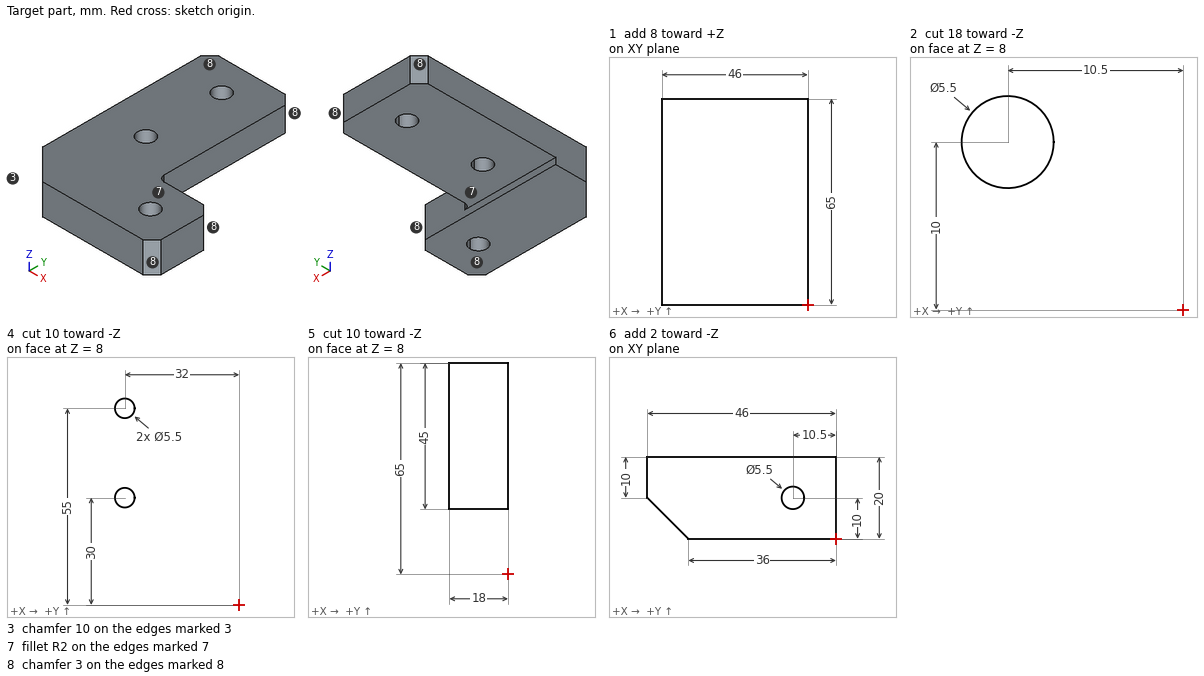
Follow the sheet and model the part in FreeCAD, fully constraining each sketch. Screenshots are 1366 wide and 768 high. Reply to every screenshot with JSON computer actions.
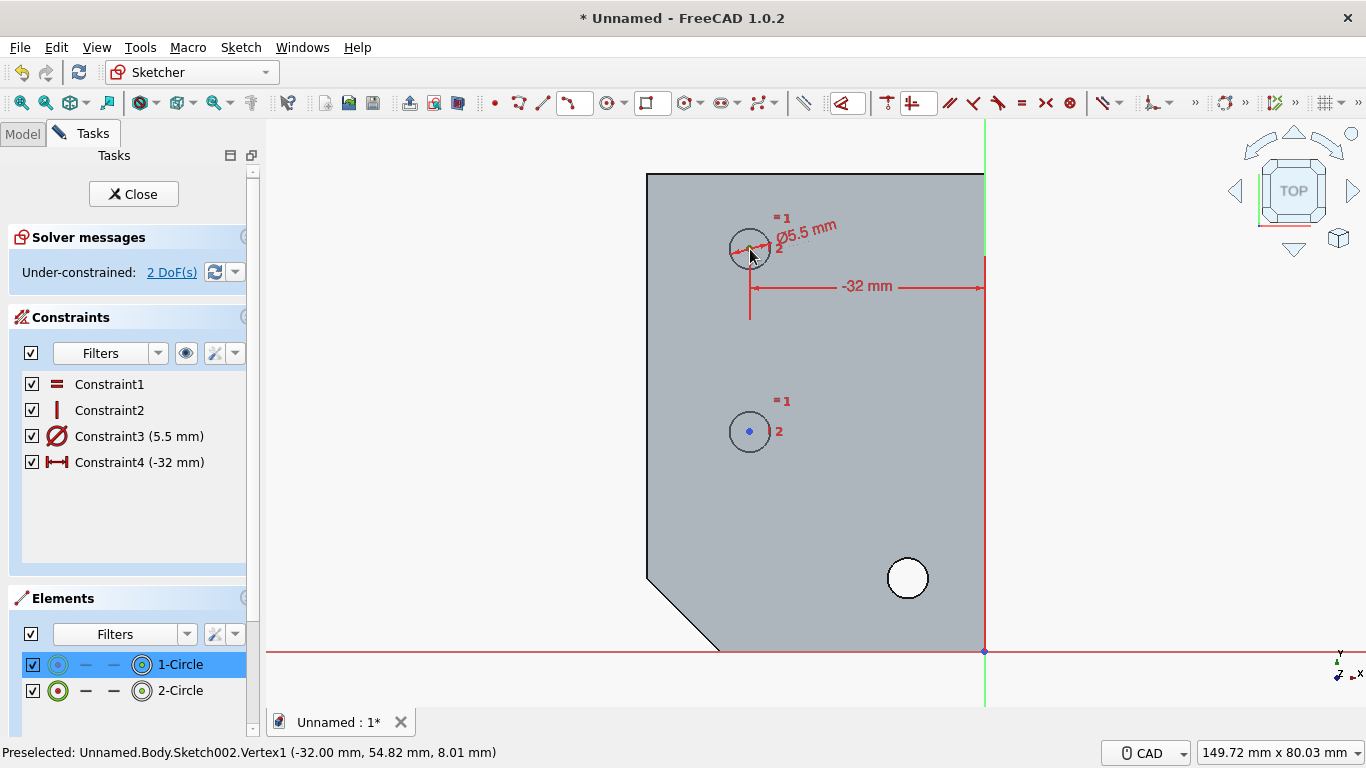
{"action": "left_click", "coordinate": [860, 104]}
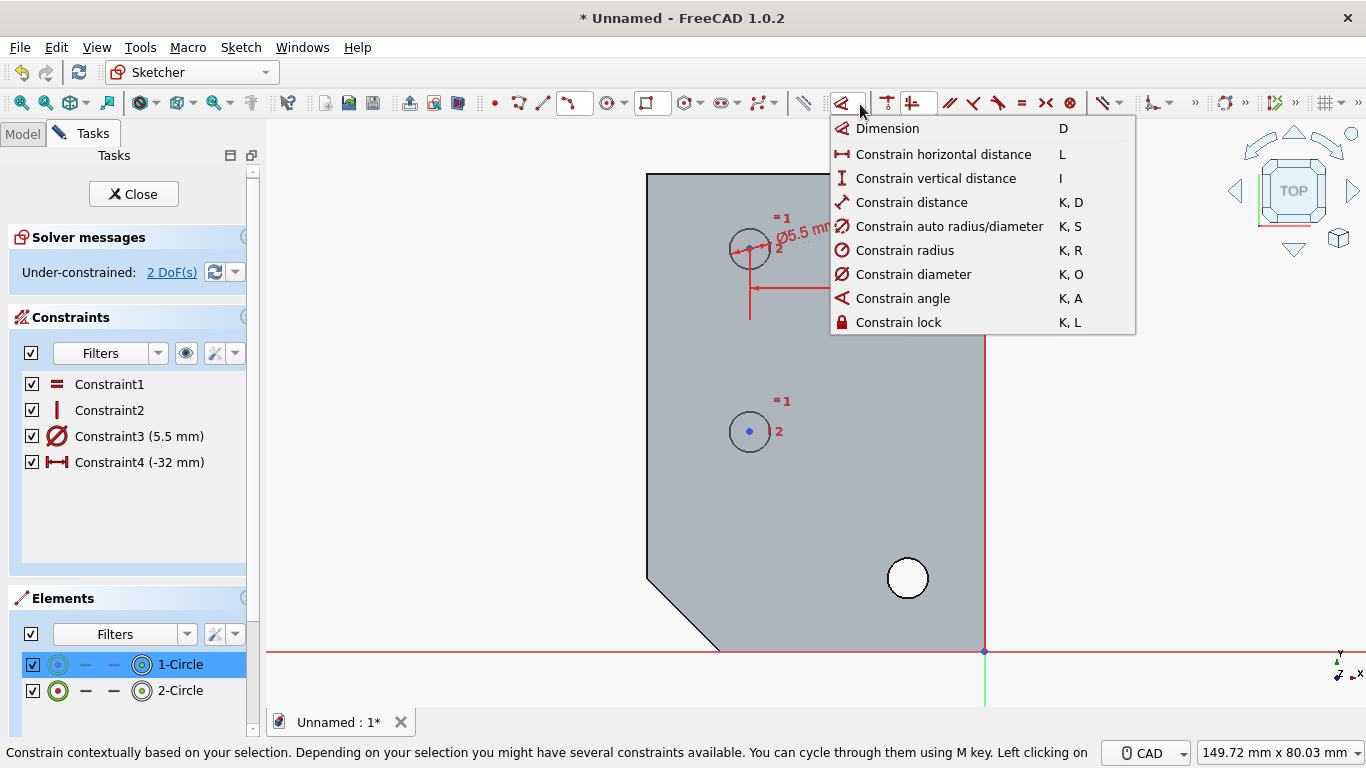
{"action": "left_click", "coordinate": [983, 178]}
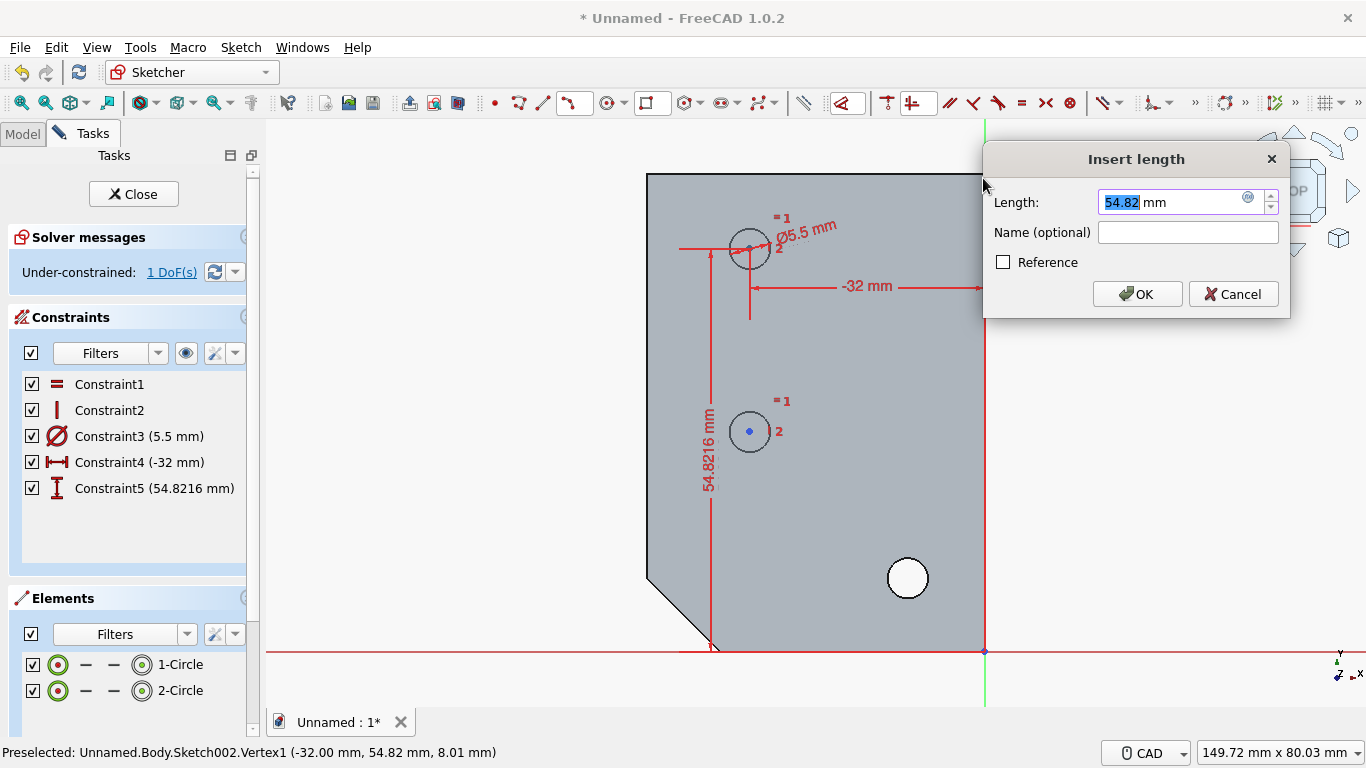
{"action": "type", "text": "55"}
{"action": "key", "text": "Return"}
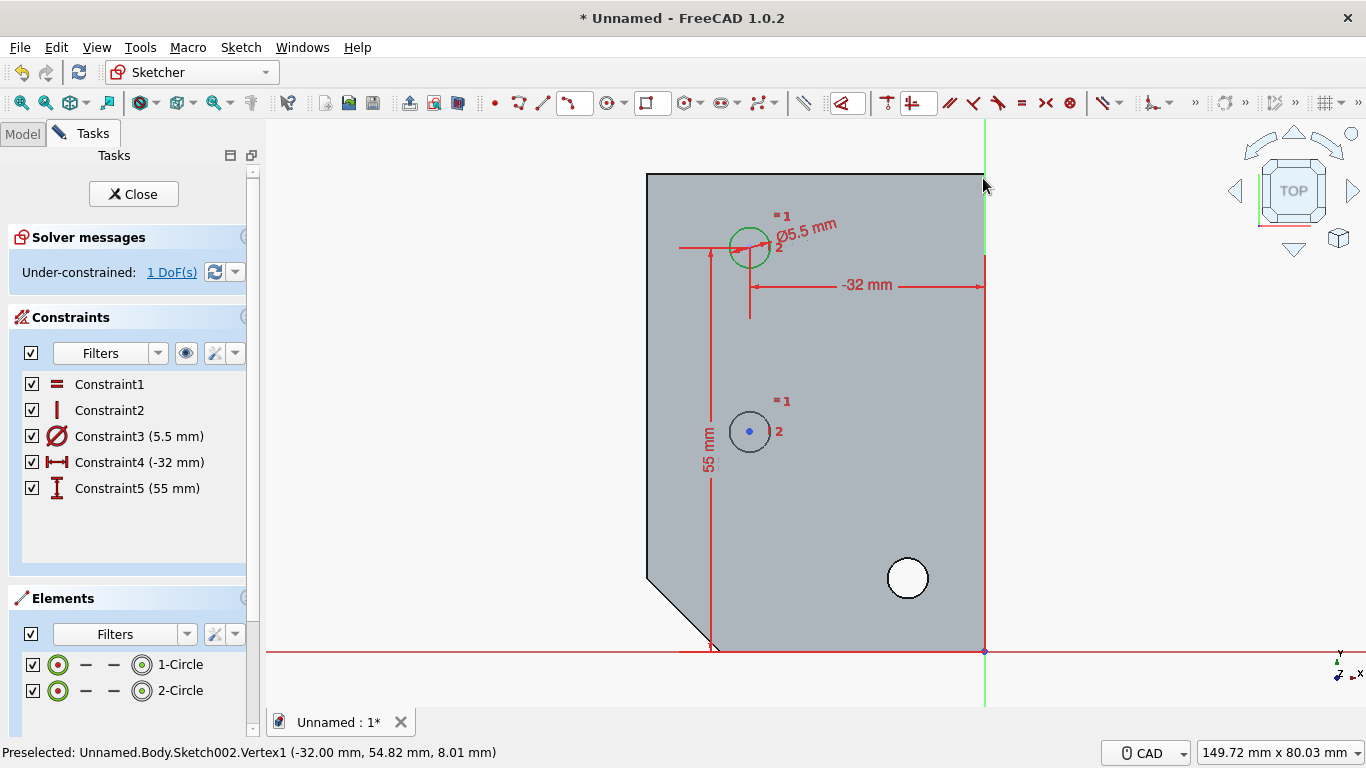
{"action": "left_click", "coordinate": [750, 432]}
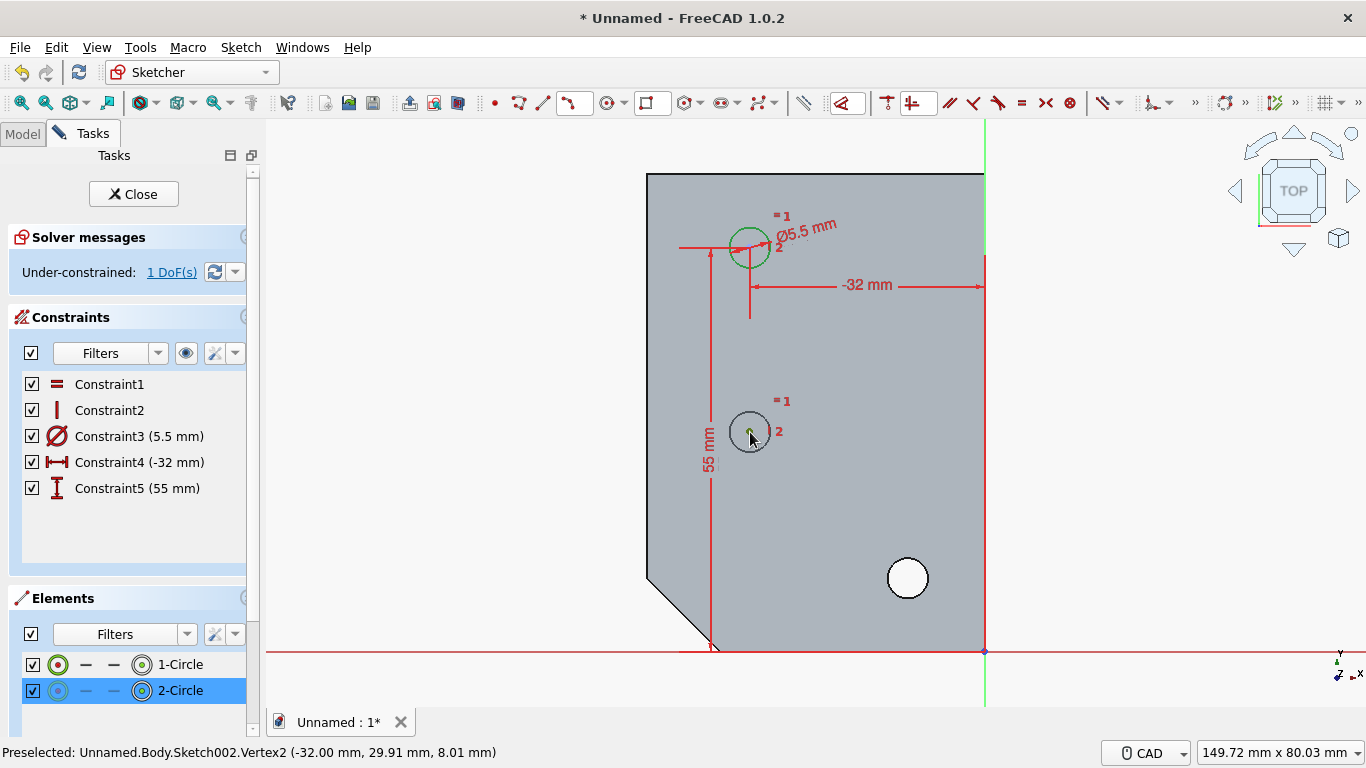
{"action": "key", "text": "i"}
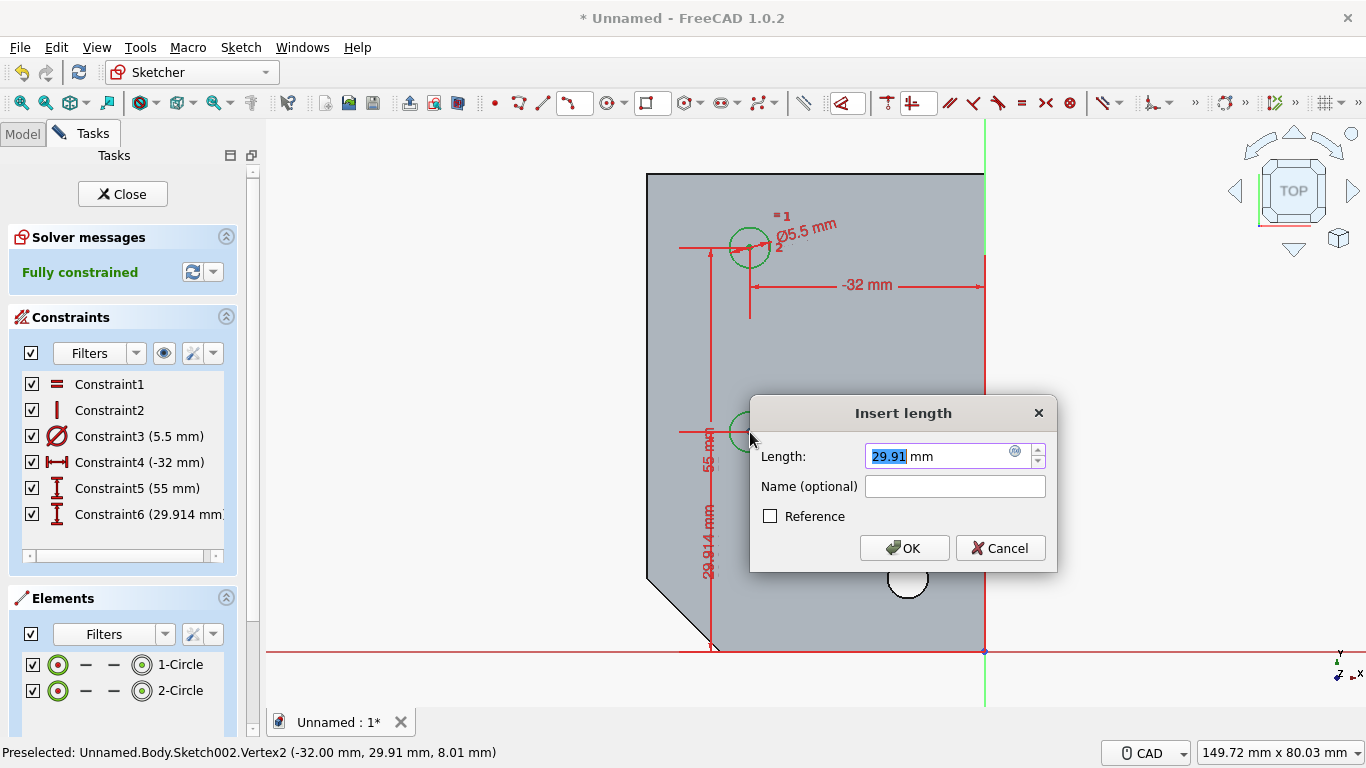
{"action": "type", "text": "30"}
{"action": "key", "text": "Return"}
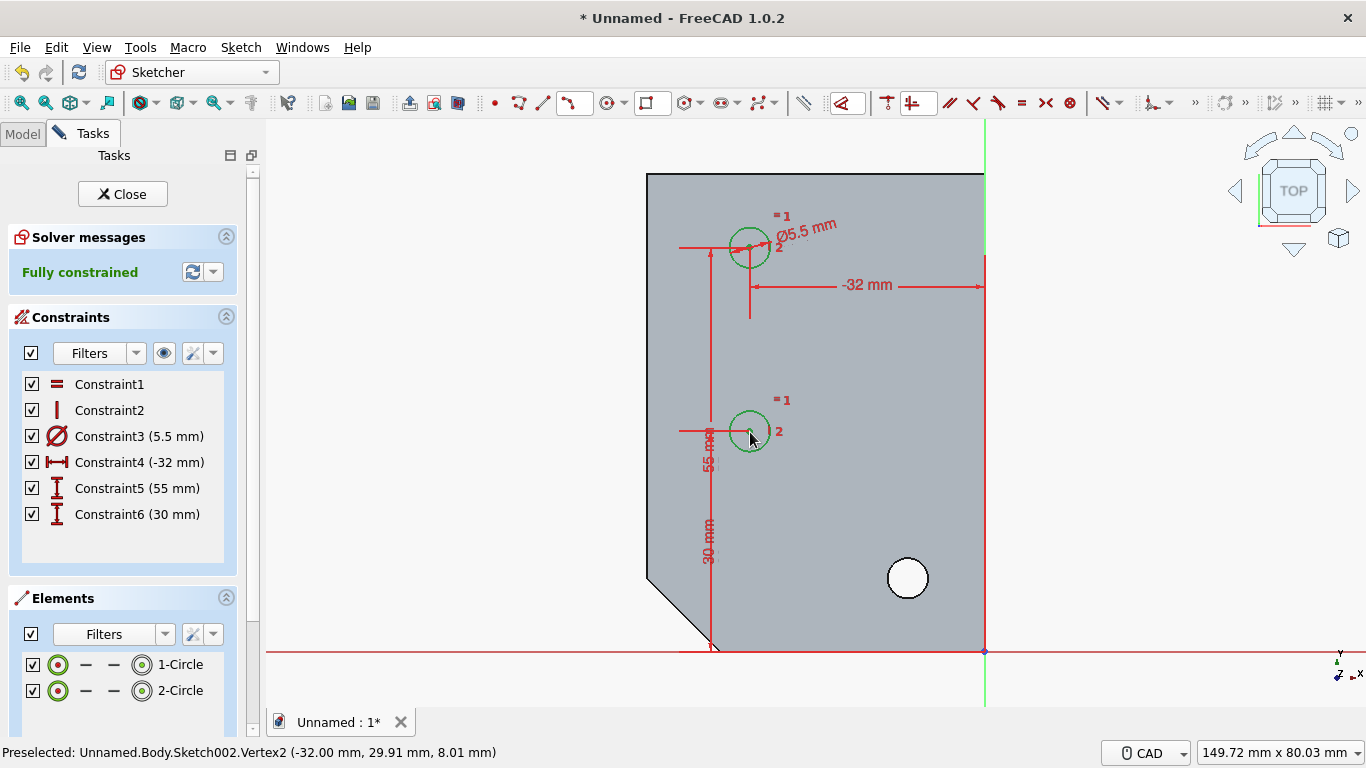
{"action": "left_click", "coordinate": [123, 194]}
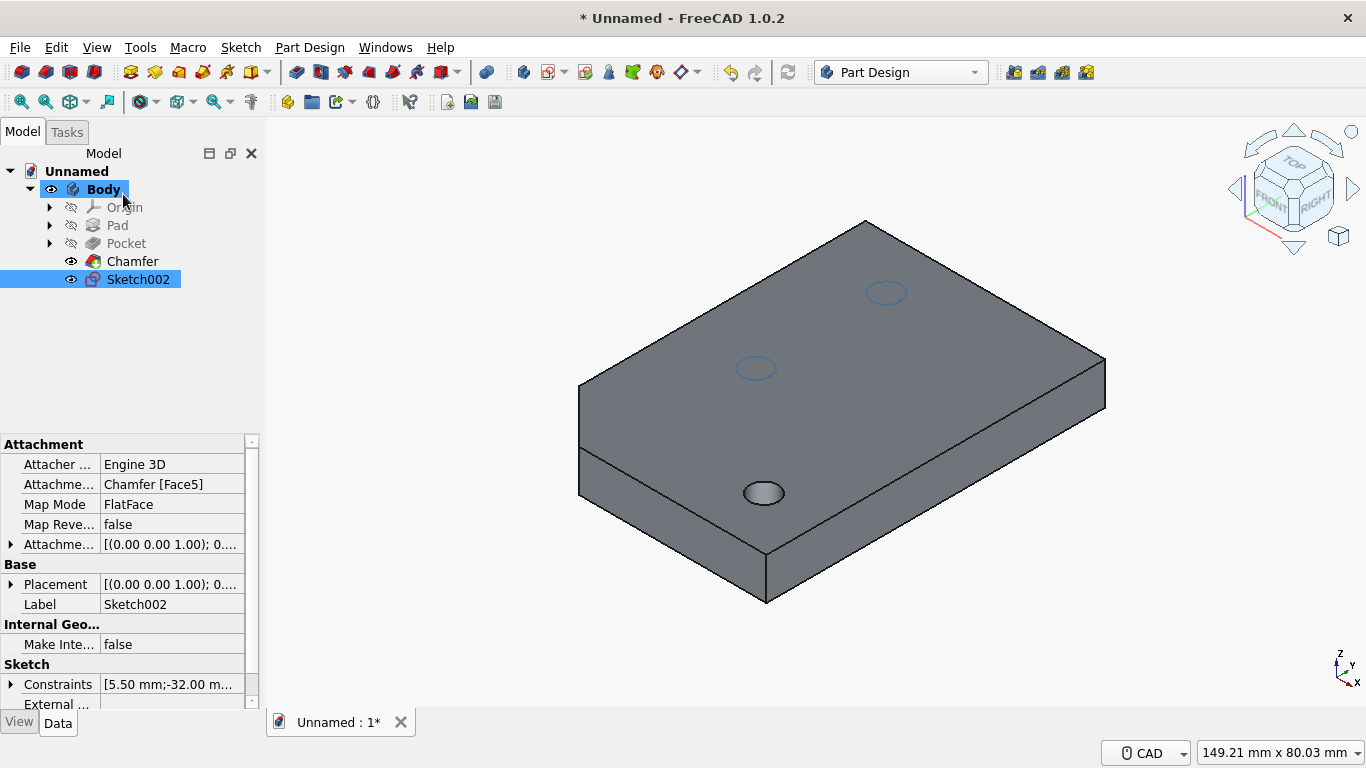
{"action": "left_click", "coordinate": [298, 72]}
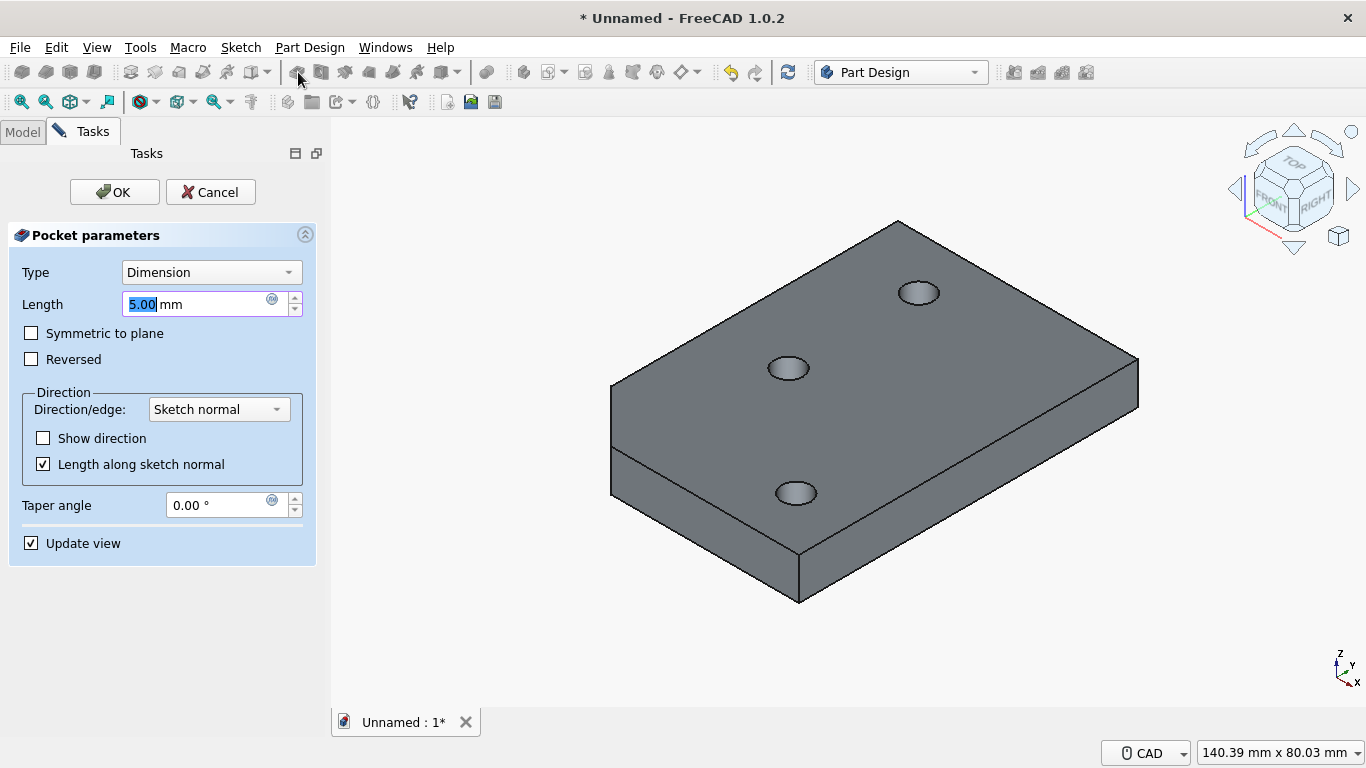
{"action": "type", "text": "10"}
{"action": "key", "text": "Tab"}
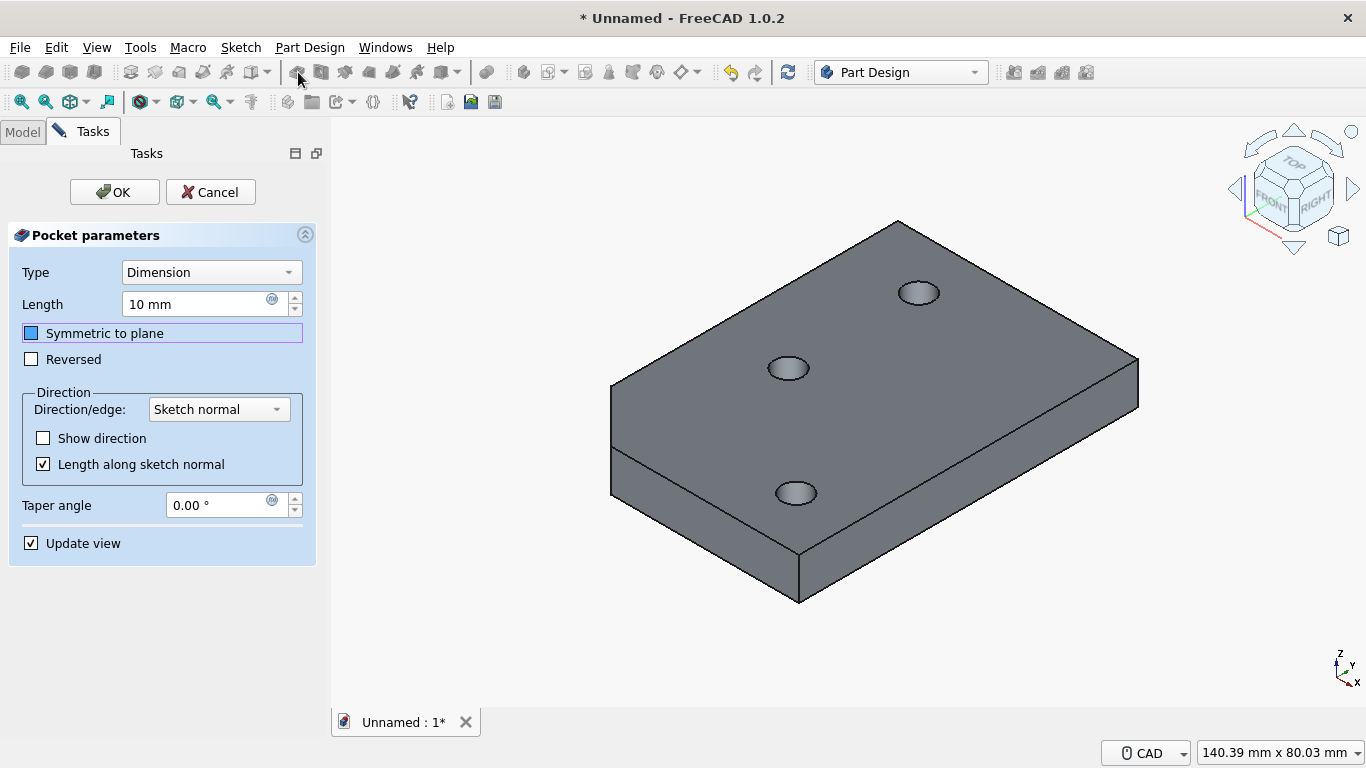
{"action": "left_click", "coordinate": [115, 192]}